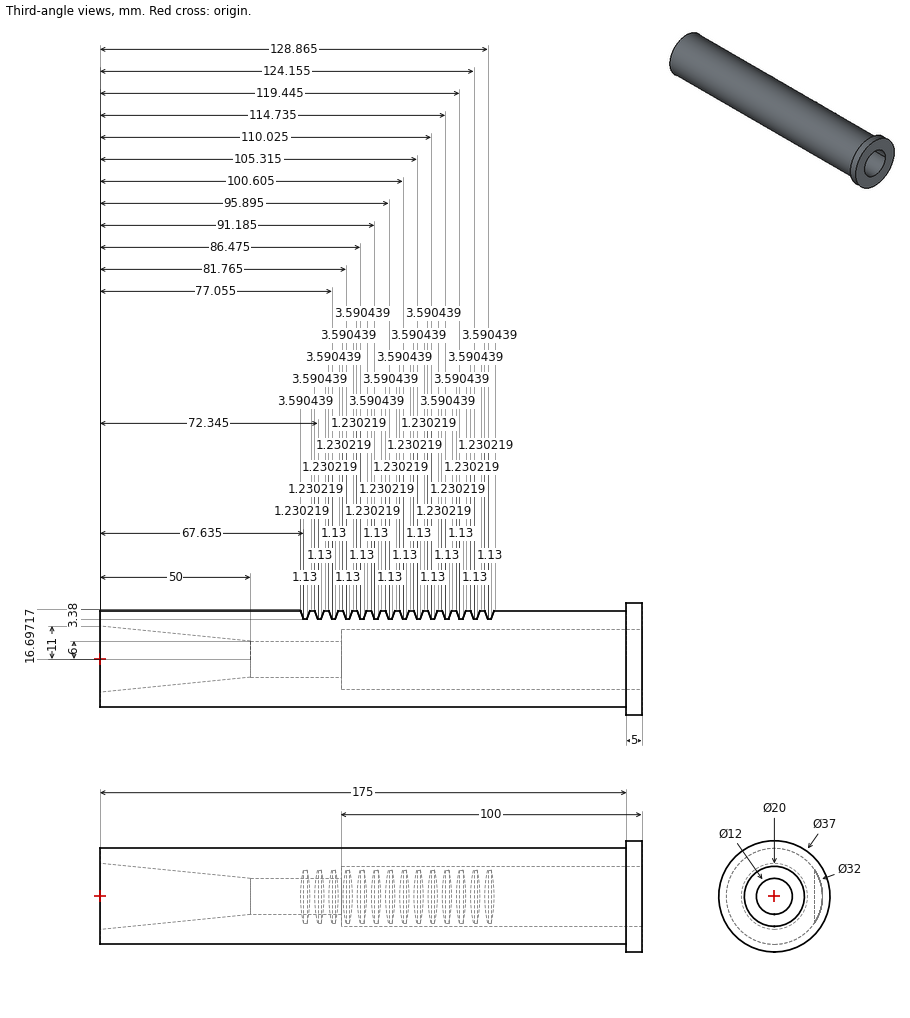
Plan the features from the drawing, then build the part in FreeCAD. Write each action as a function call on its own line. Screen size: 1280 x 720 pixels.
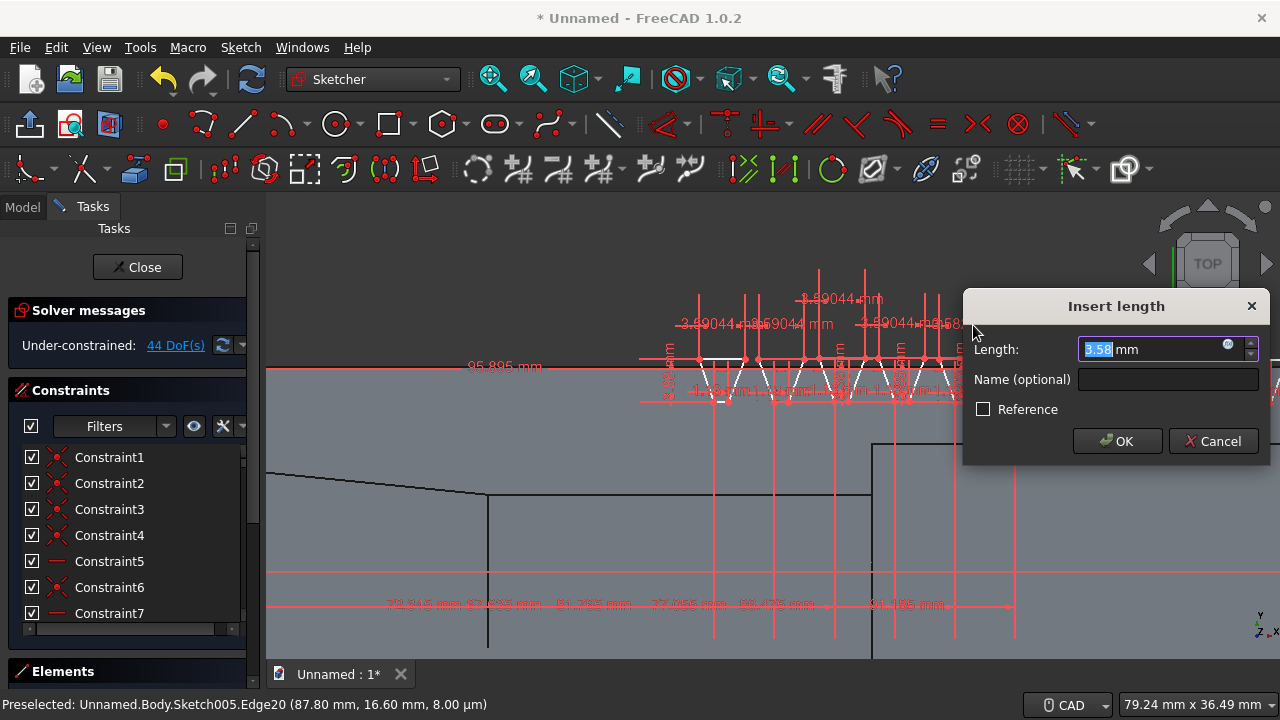
text(3.590439)
key(Return)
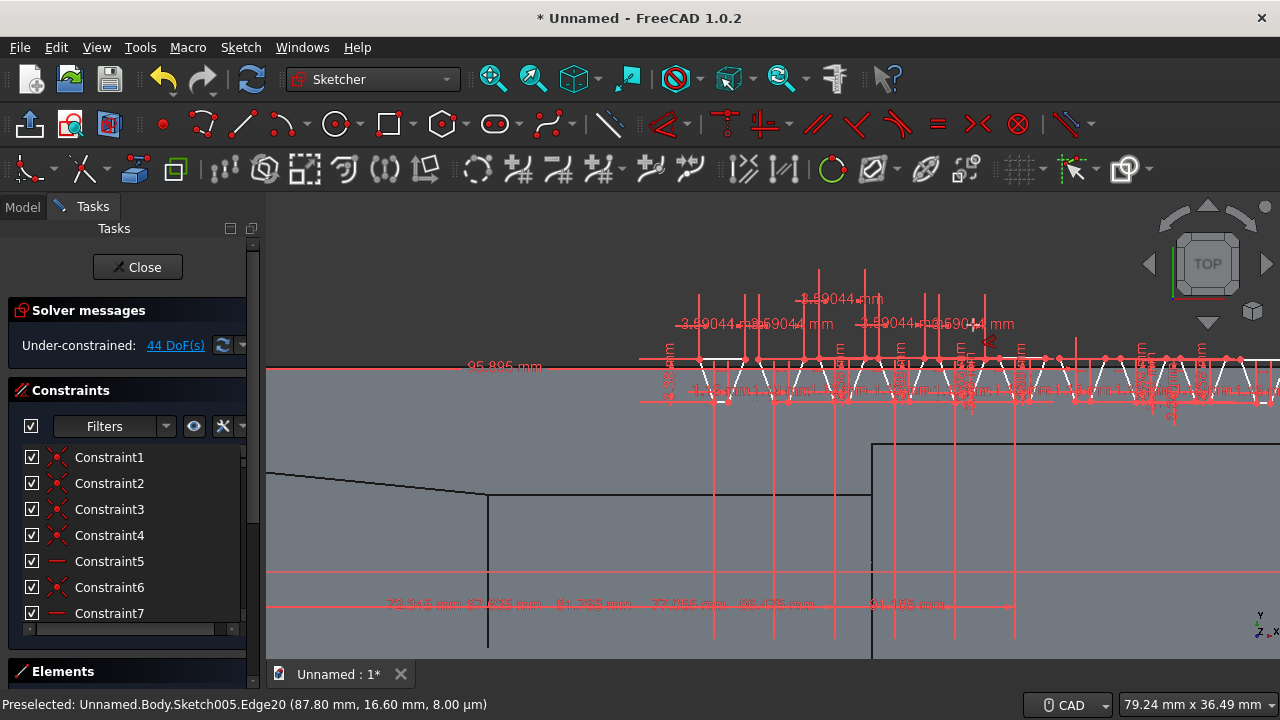
click(1032, 358)
click(1023, 300)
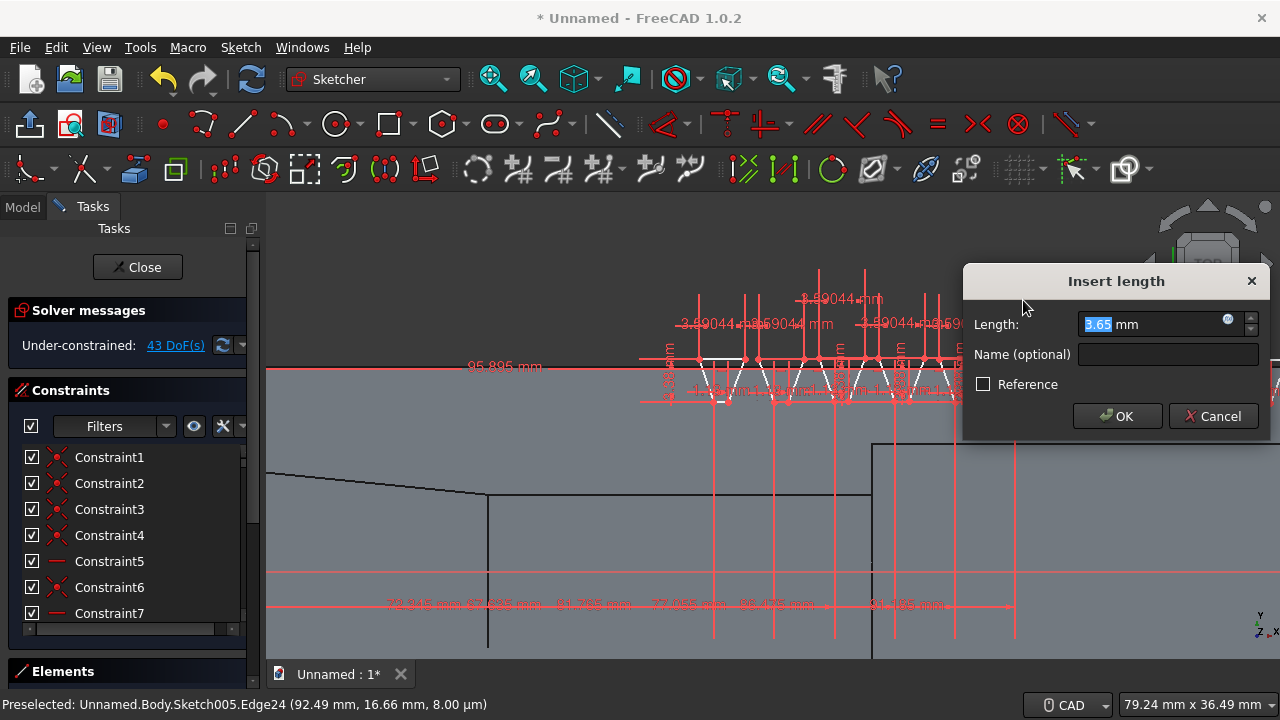
text(3.590439)
key(Return)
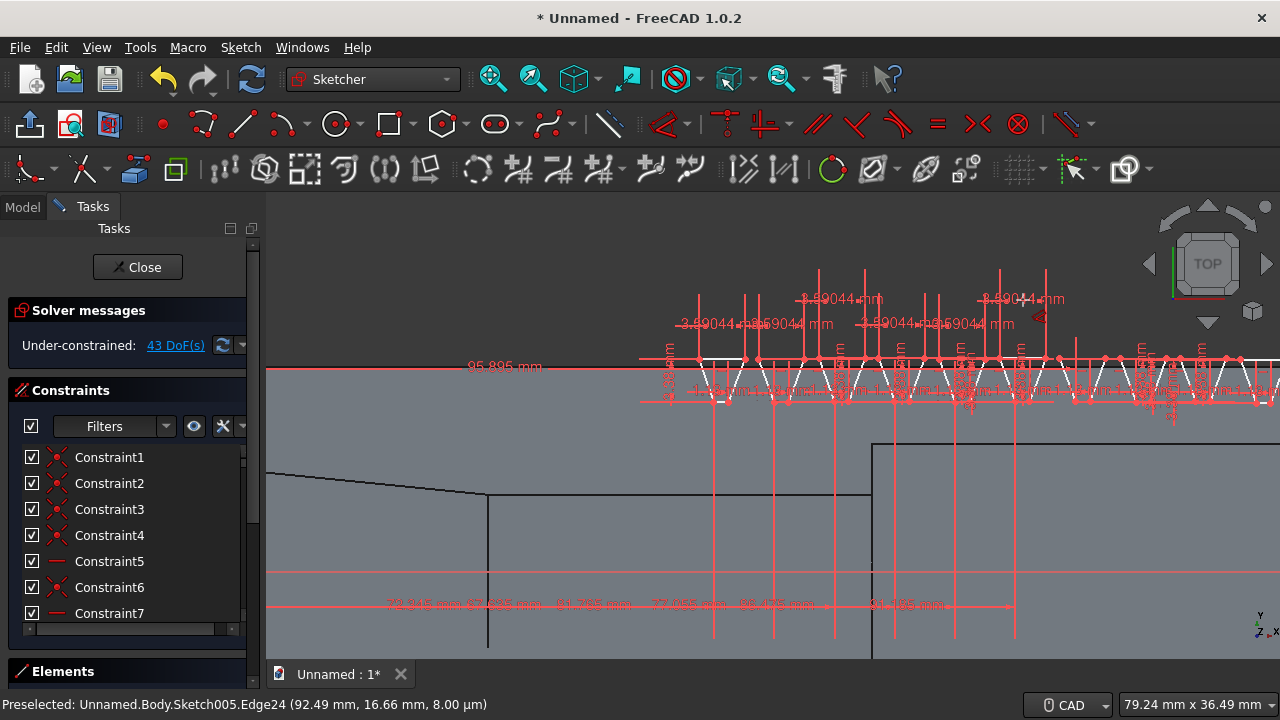
click(1092, 359)
click(1083, 325)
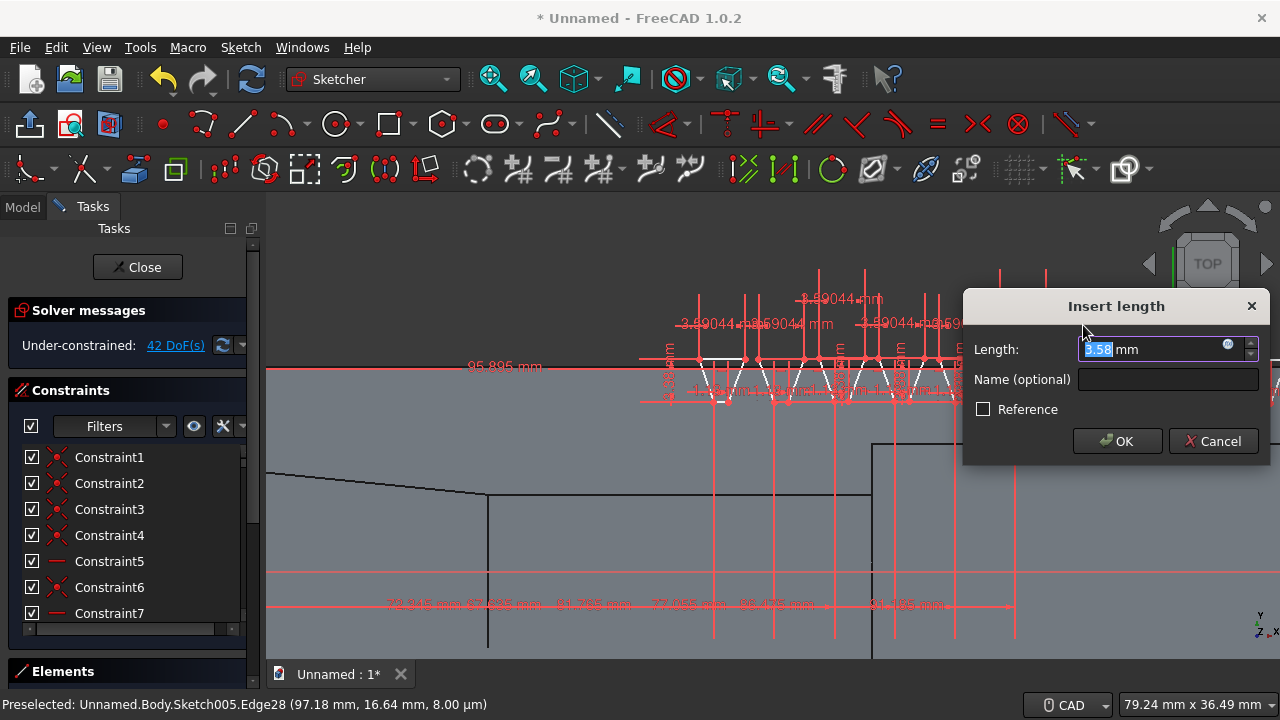
text(3.590439)
key(Return)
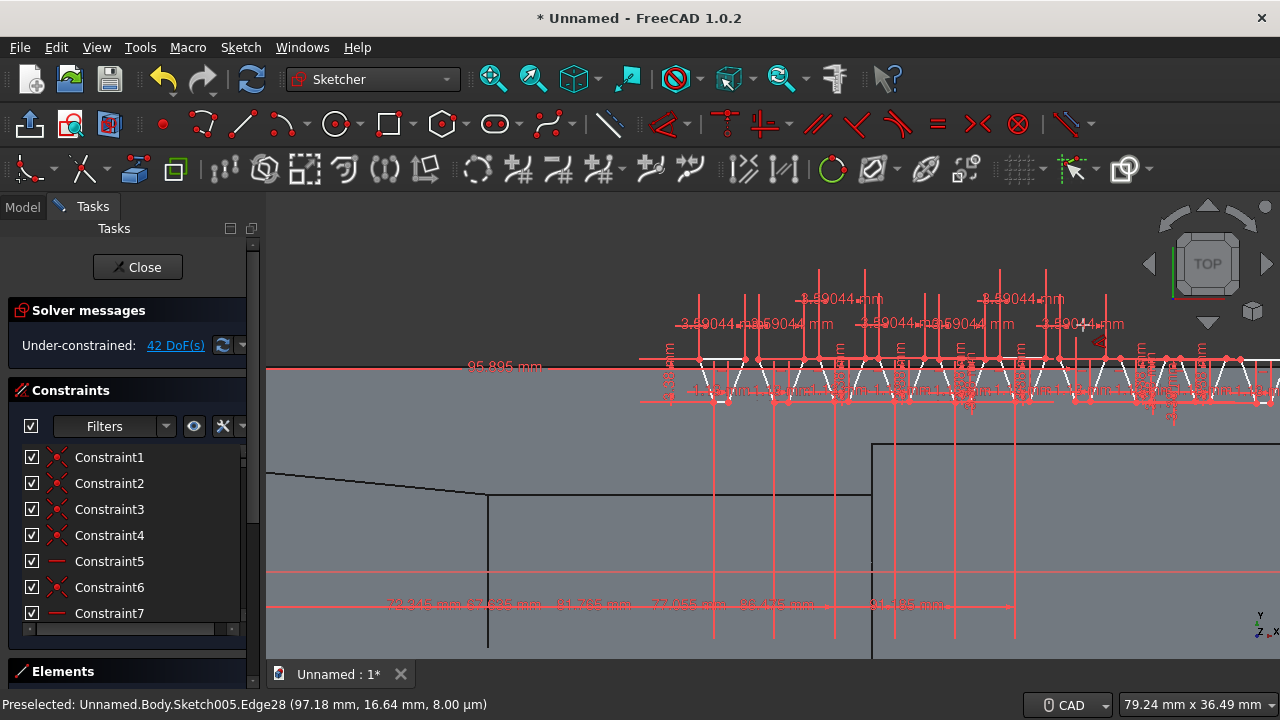
scroll(714, 403, down, 5)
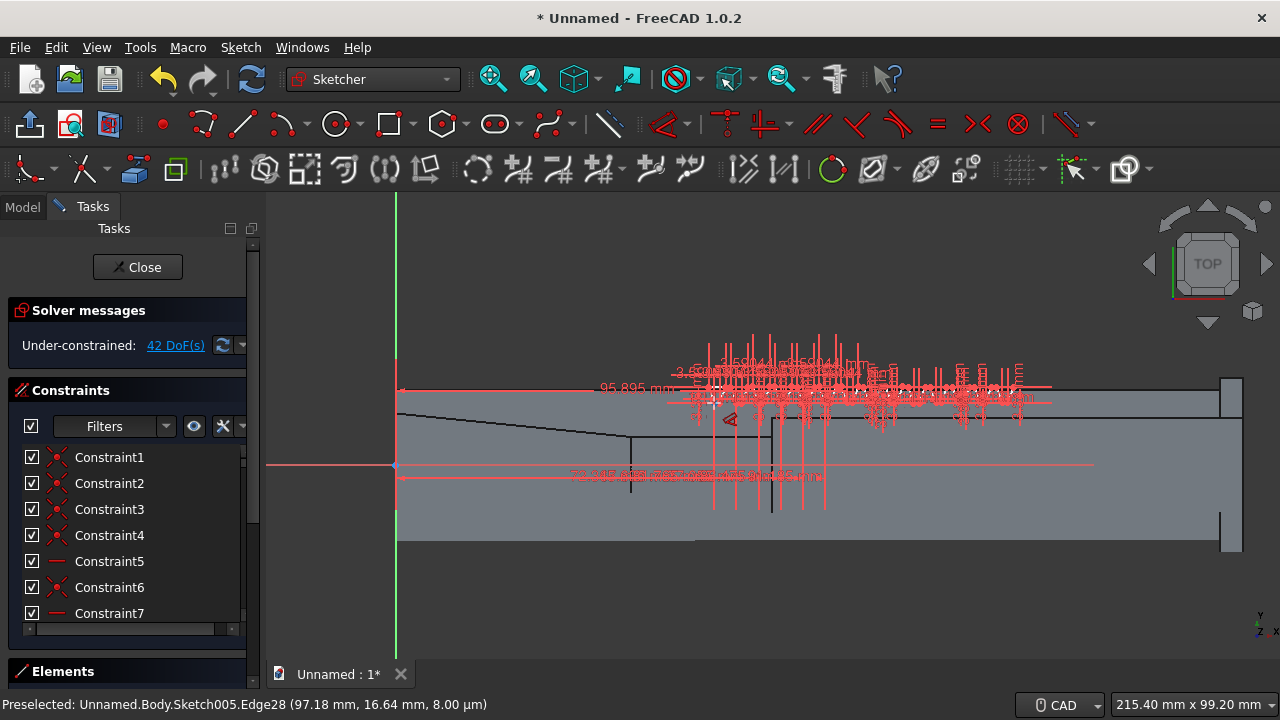
scroll(876, 387, up, 6)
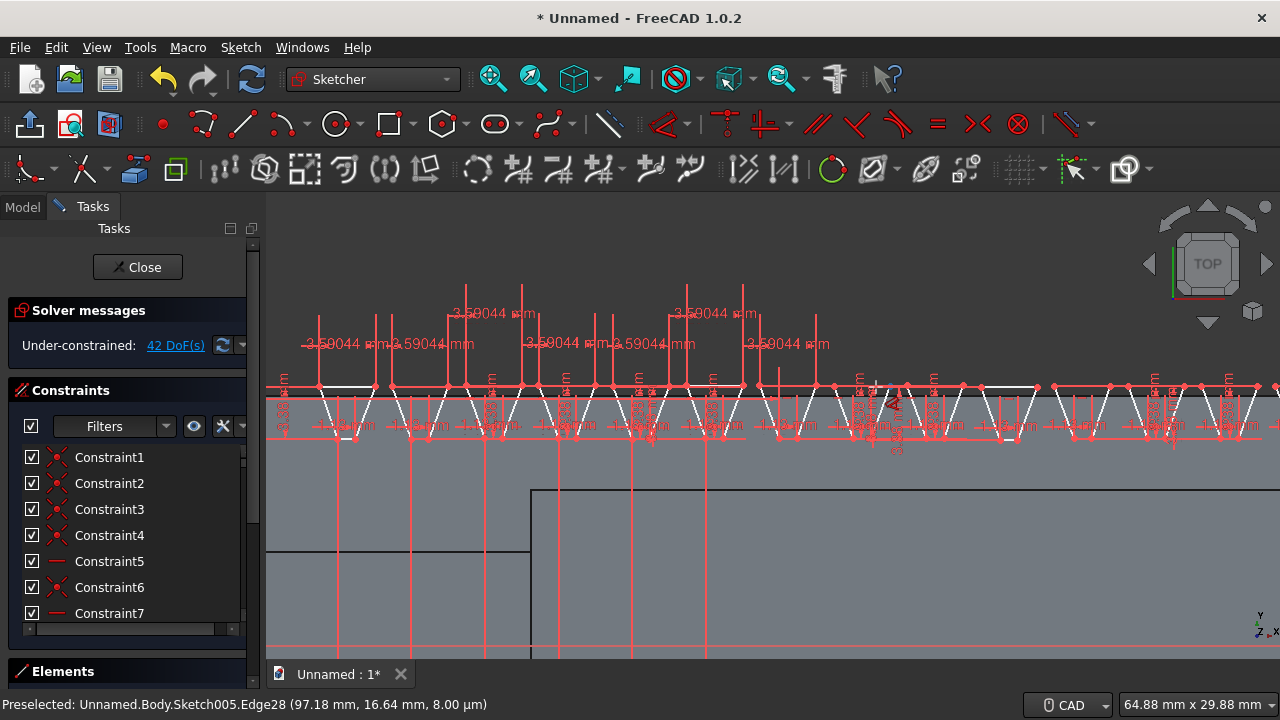
click(873, 386)
click(862, 352)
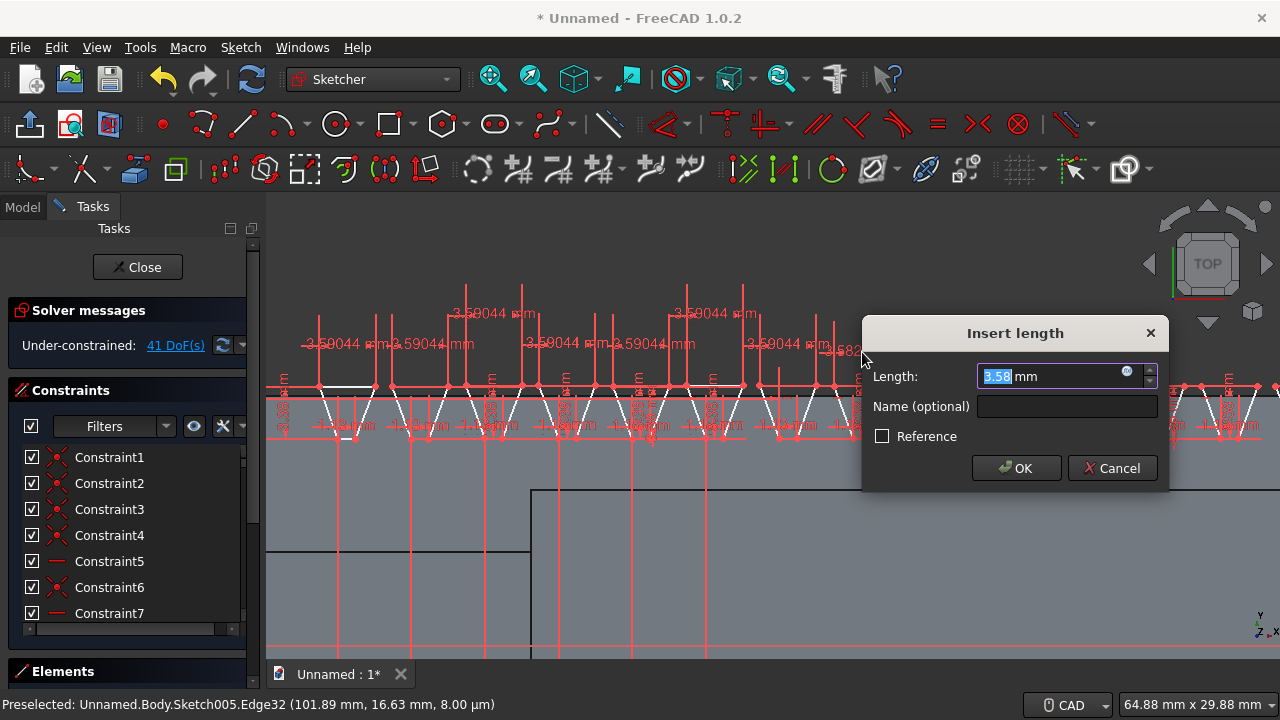
text(3.590439)
key(Return)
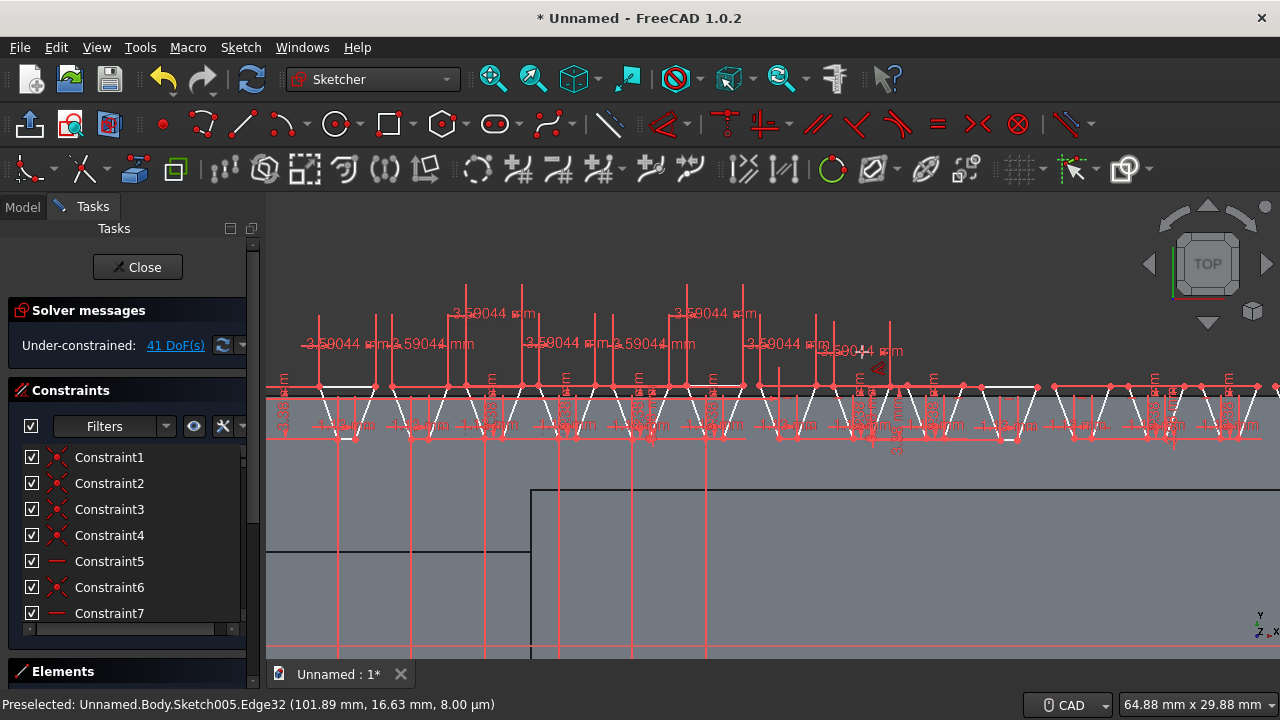
click(946, 386)
click(935, 352)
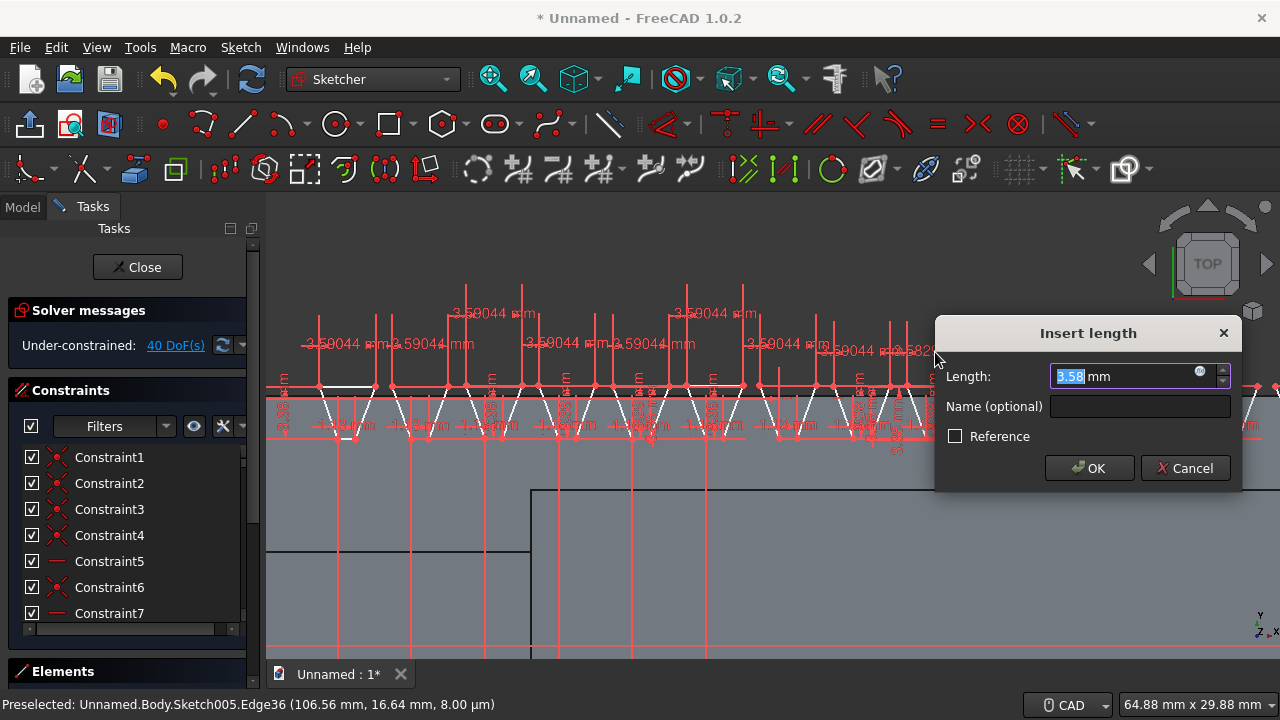
text(3.590439)
key(Return)